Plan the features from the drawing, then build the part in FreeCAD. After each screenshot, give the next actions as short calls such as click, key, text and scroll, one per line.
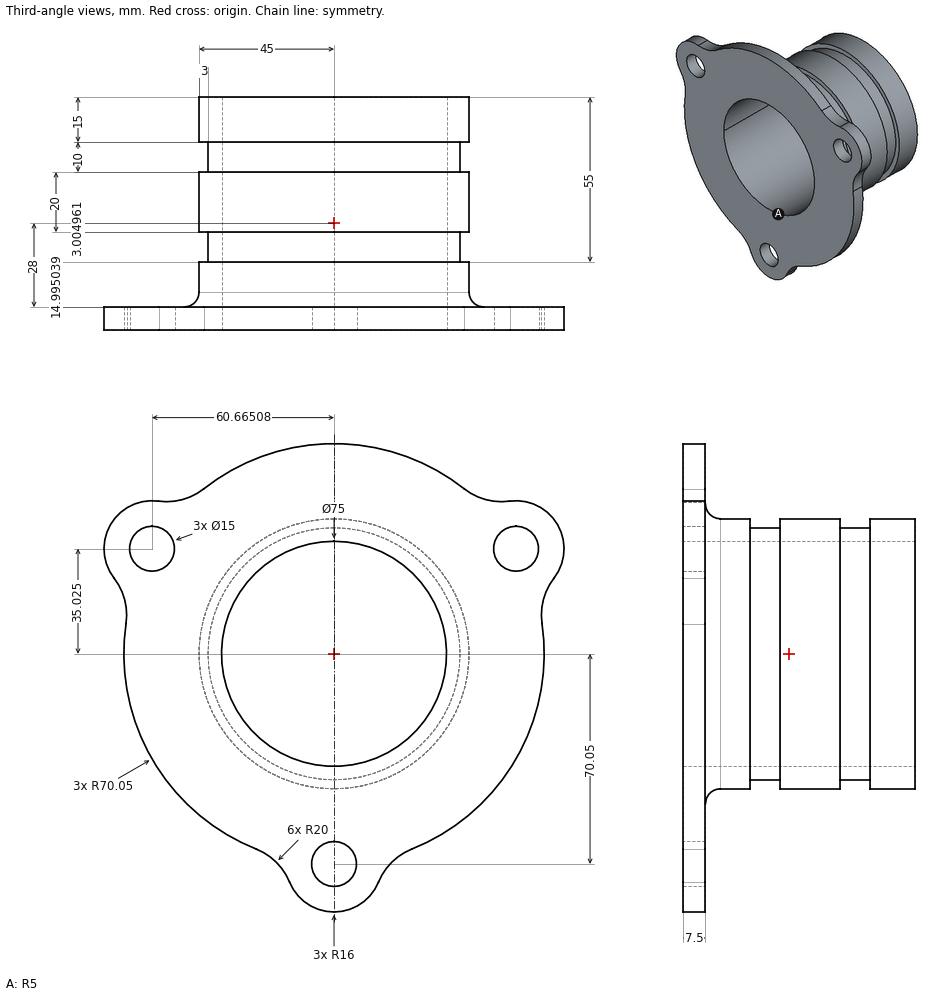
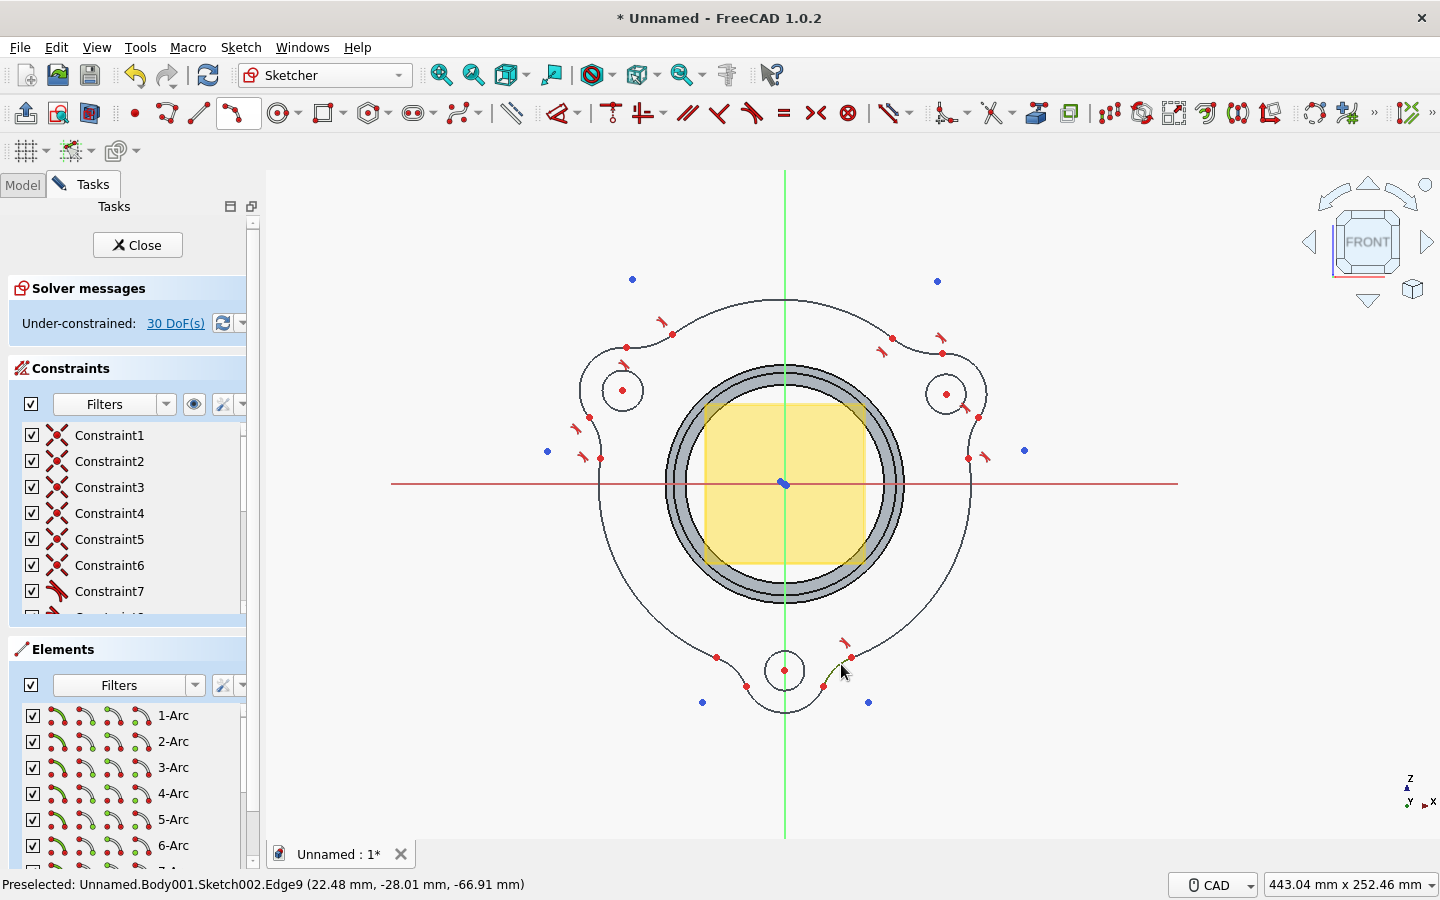
click(766, 708)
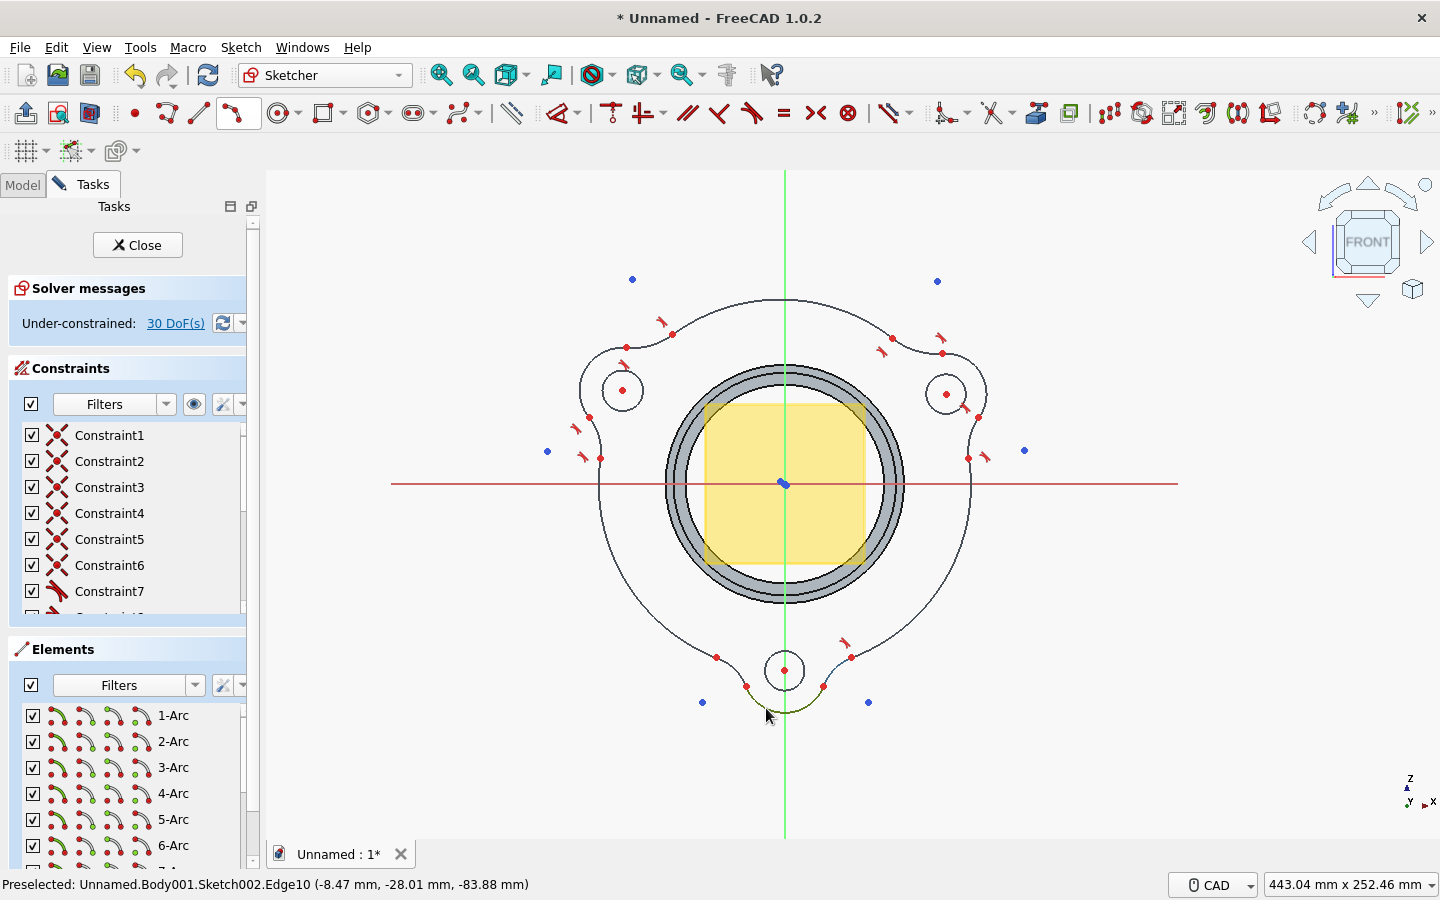
key(t)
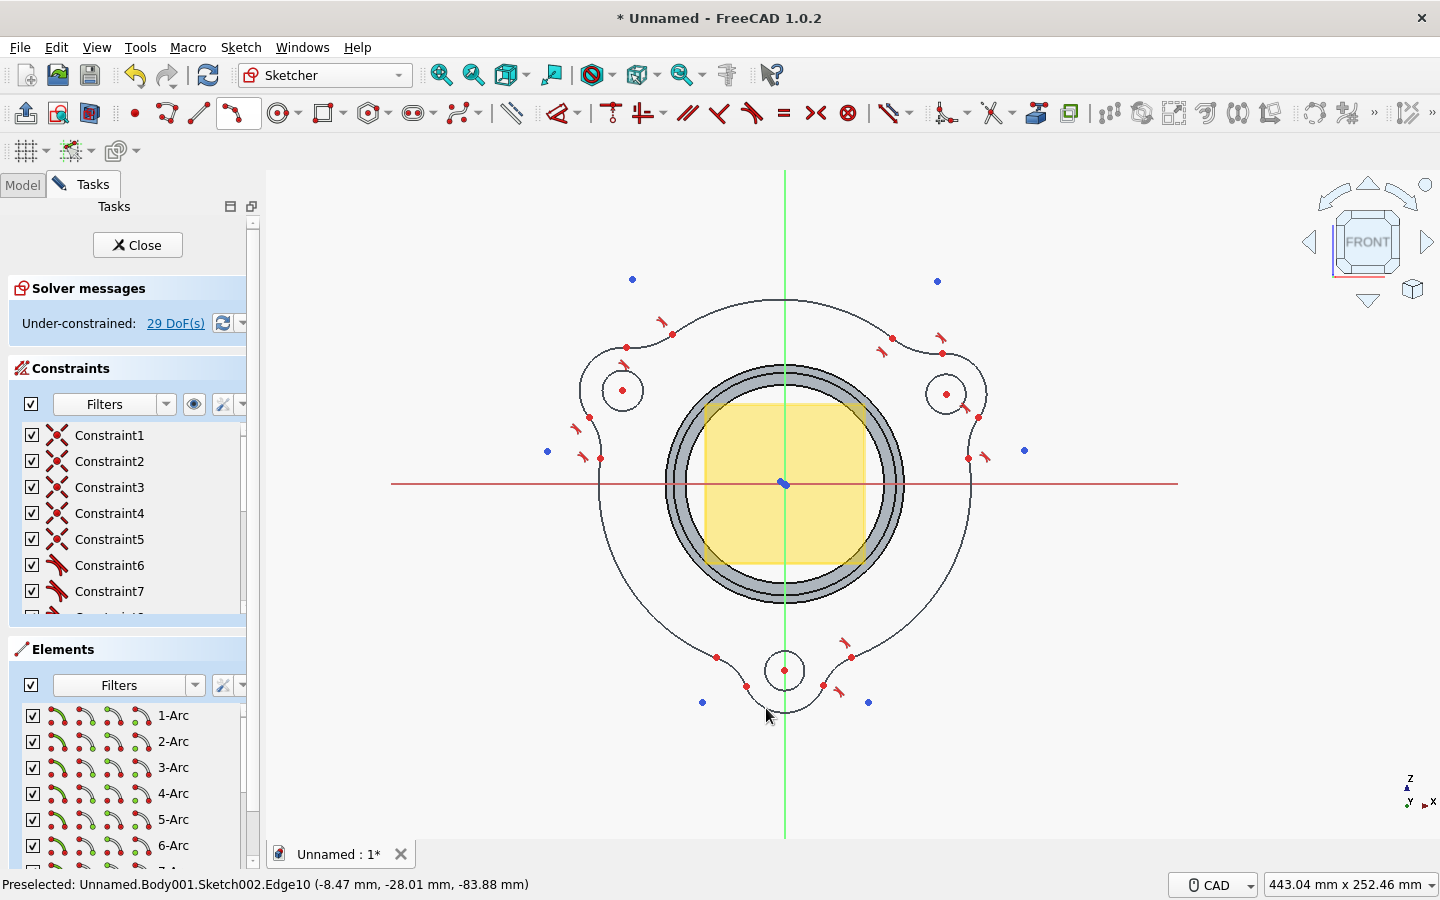
click(766, 708)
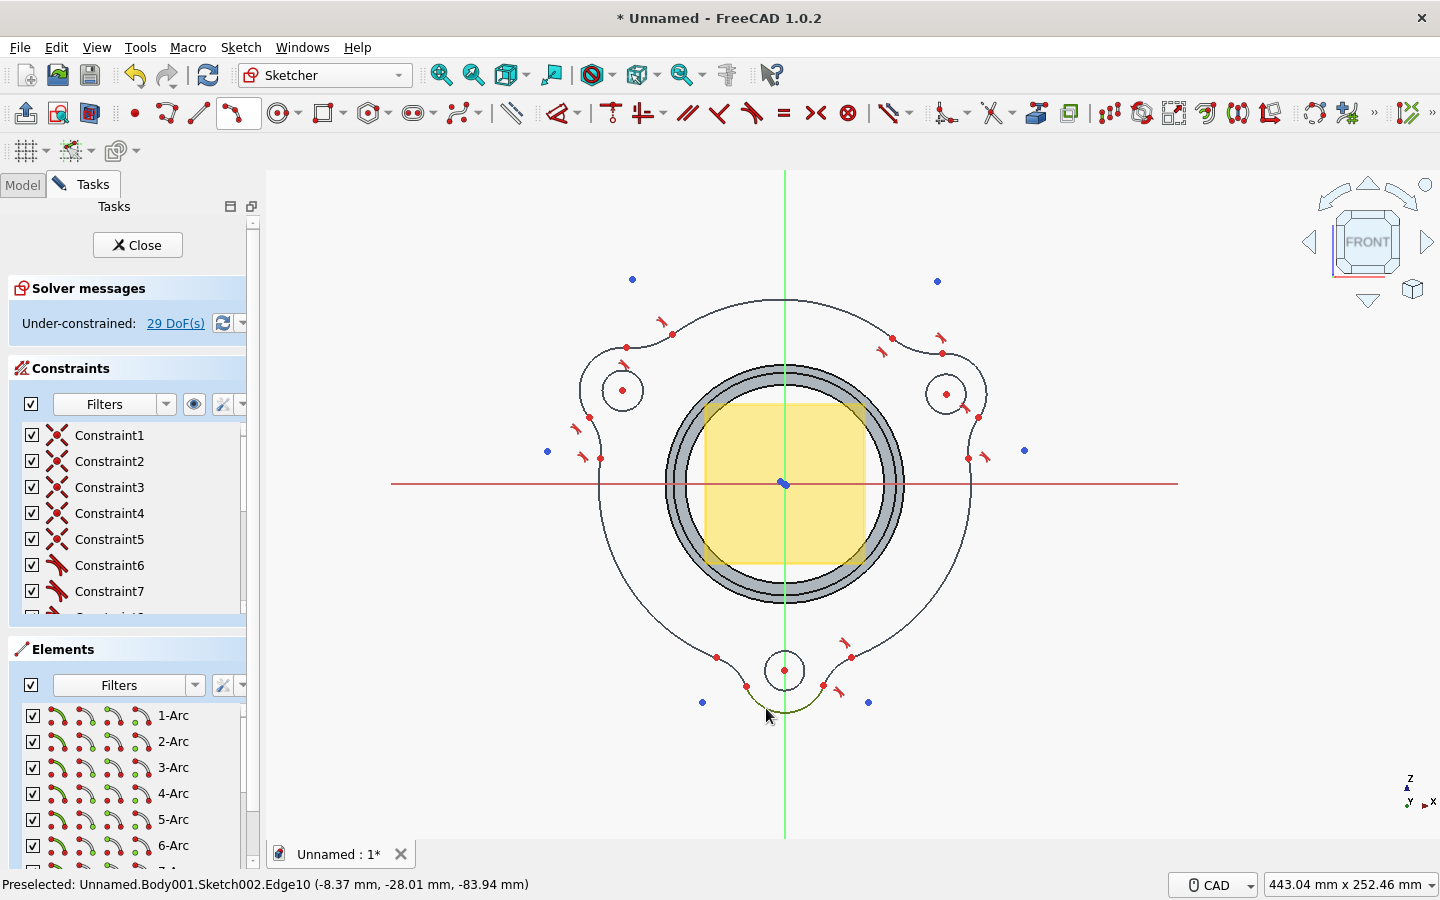
click(740, 675)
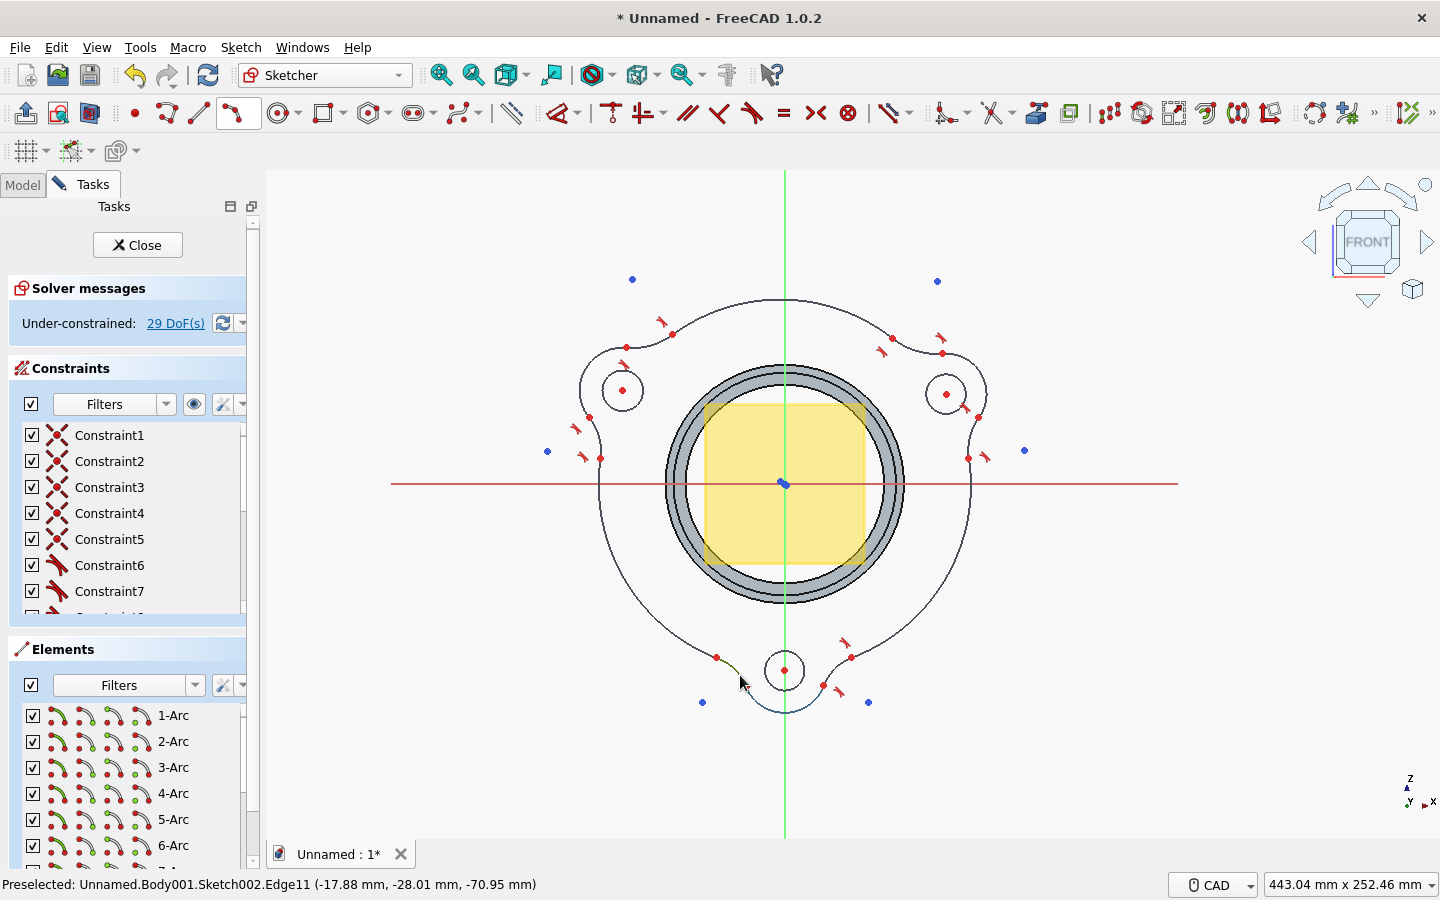
click(752, 114)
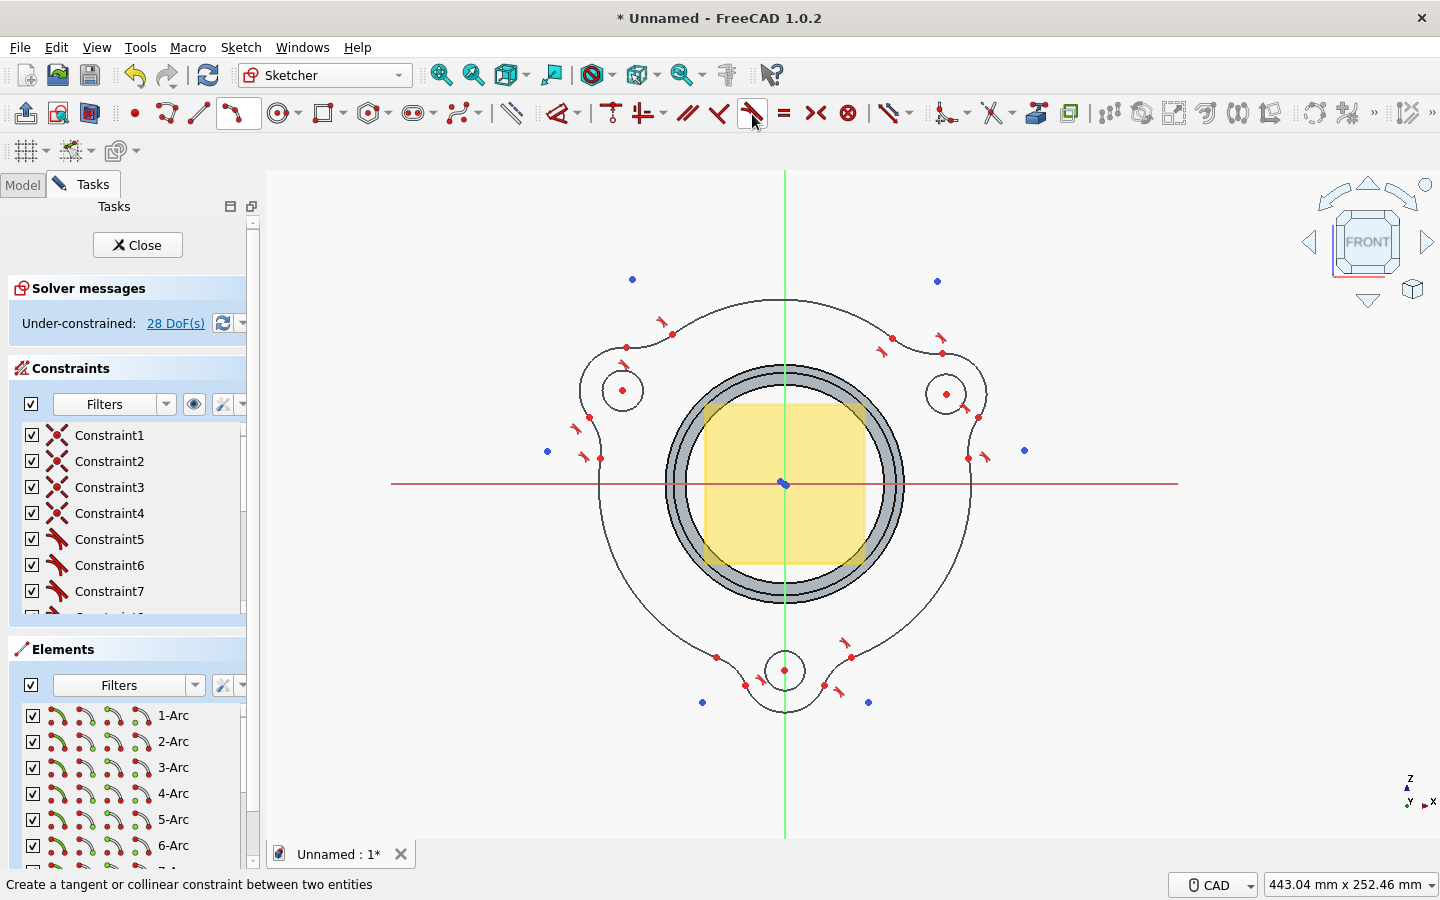
click(740, 674)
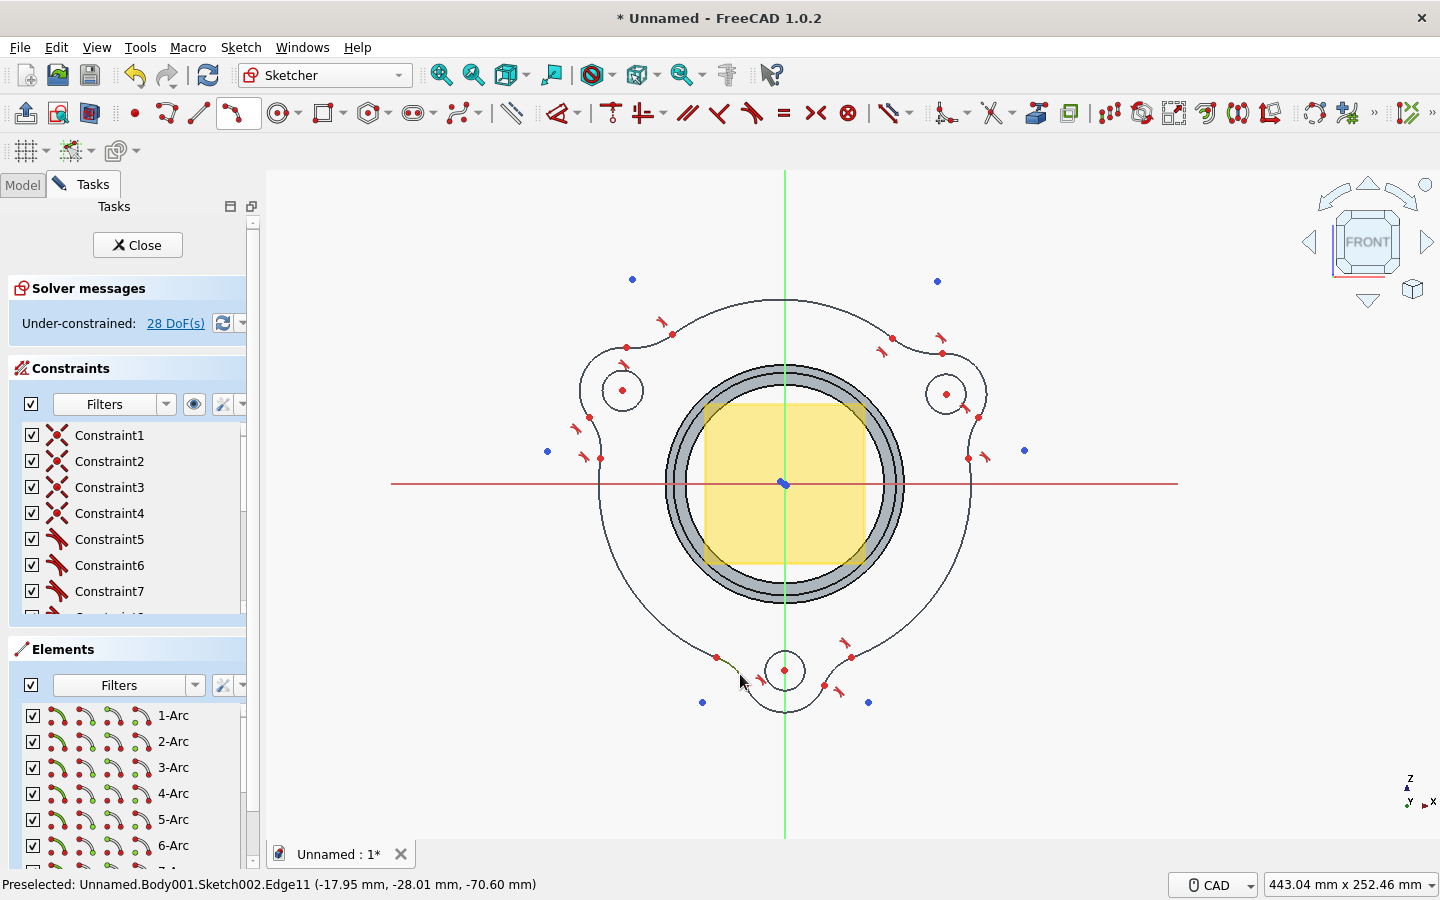
click(605, 532)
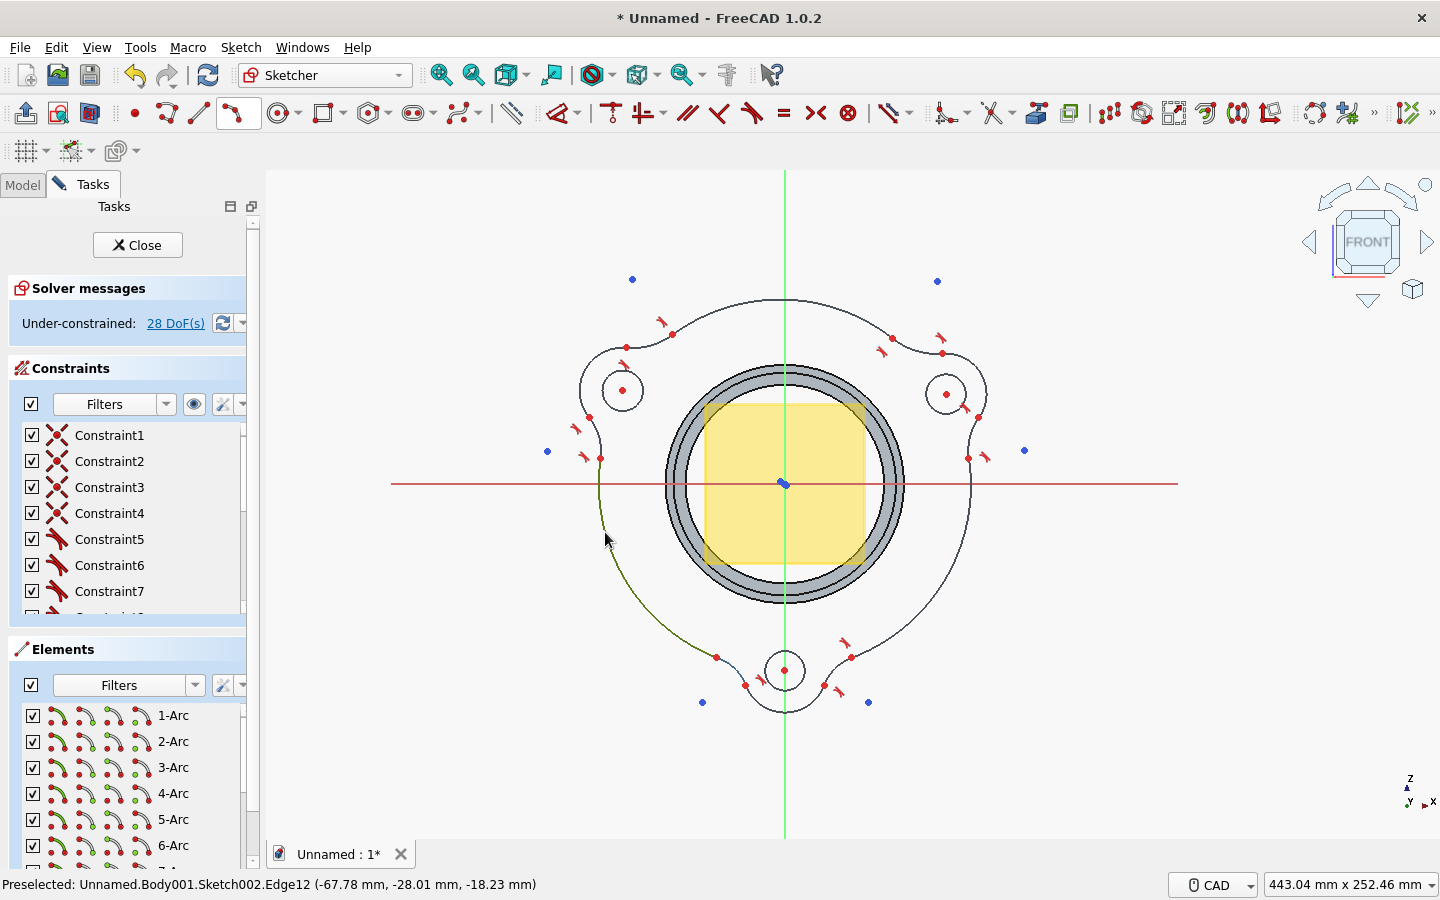
key(t)